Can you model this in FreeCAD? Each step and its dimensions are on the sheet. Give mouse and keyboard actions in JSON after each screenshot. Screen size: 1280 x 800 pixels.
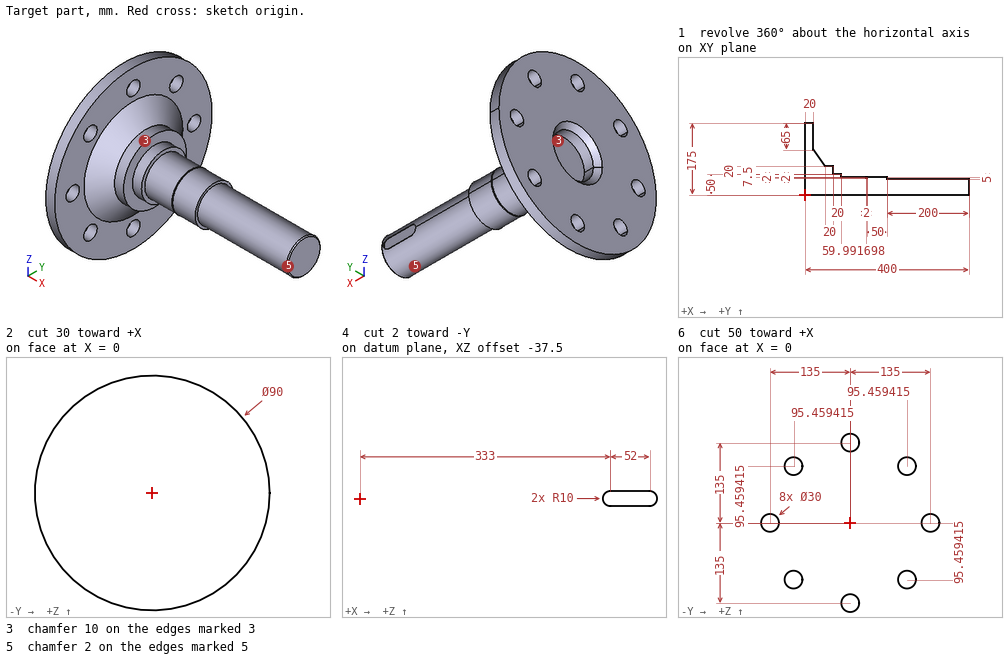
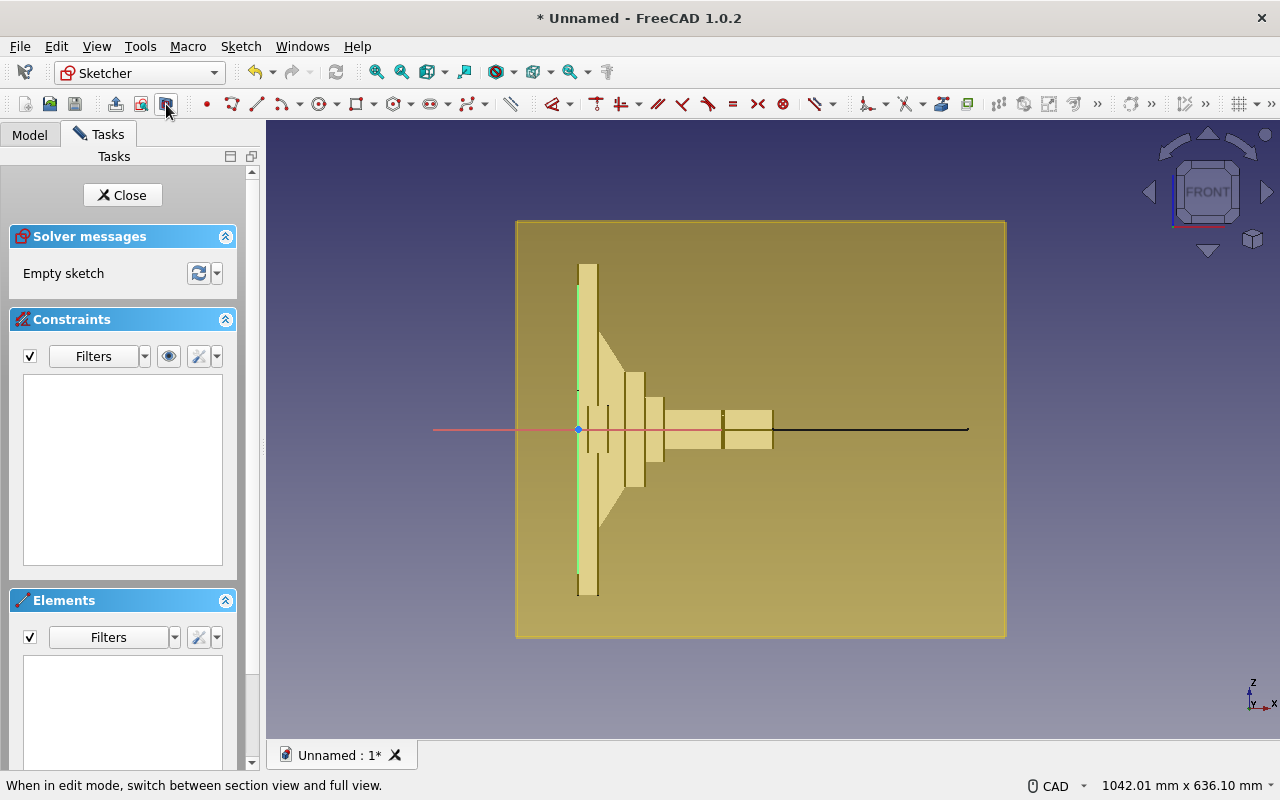
{"action": "scroll", "coordinate": [956, 430], "scroll_direction": "up", "scroll_amount": 11}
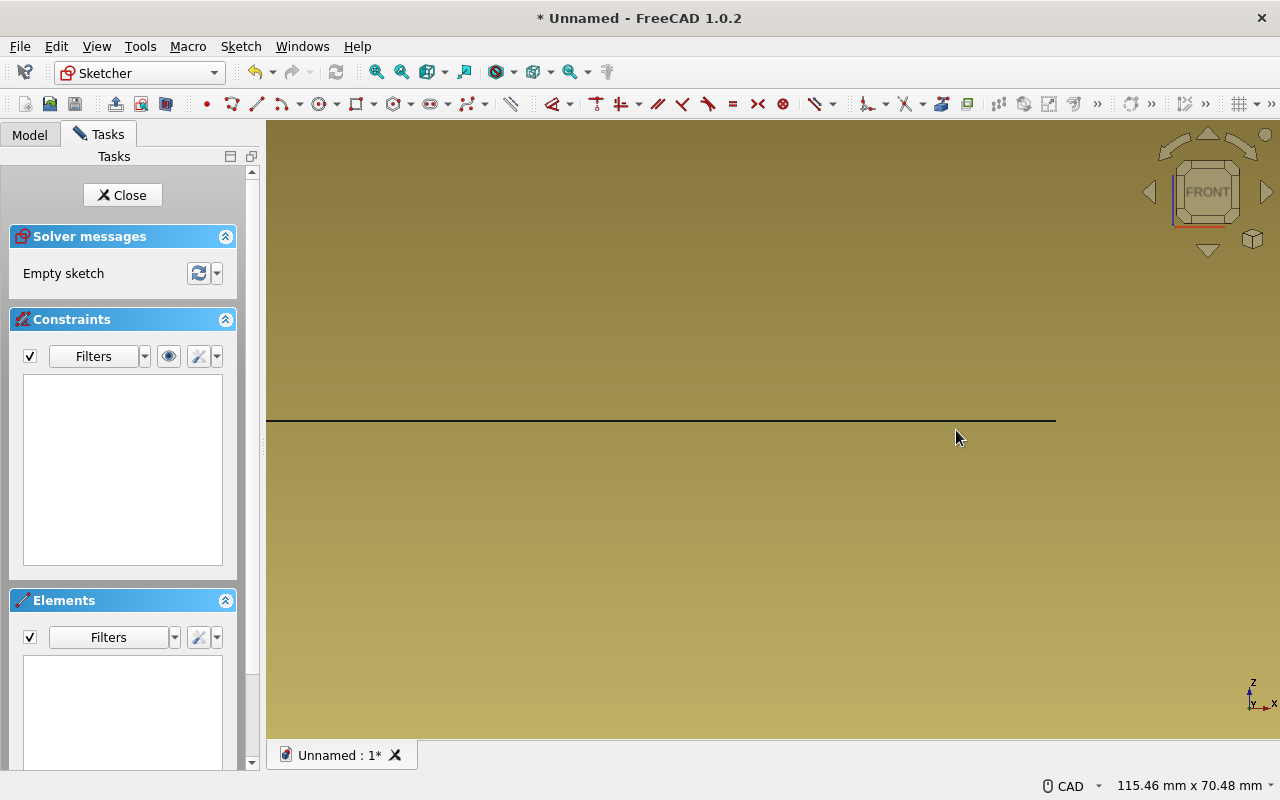
{"action": "left_click", "coordinate": [430, 104]}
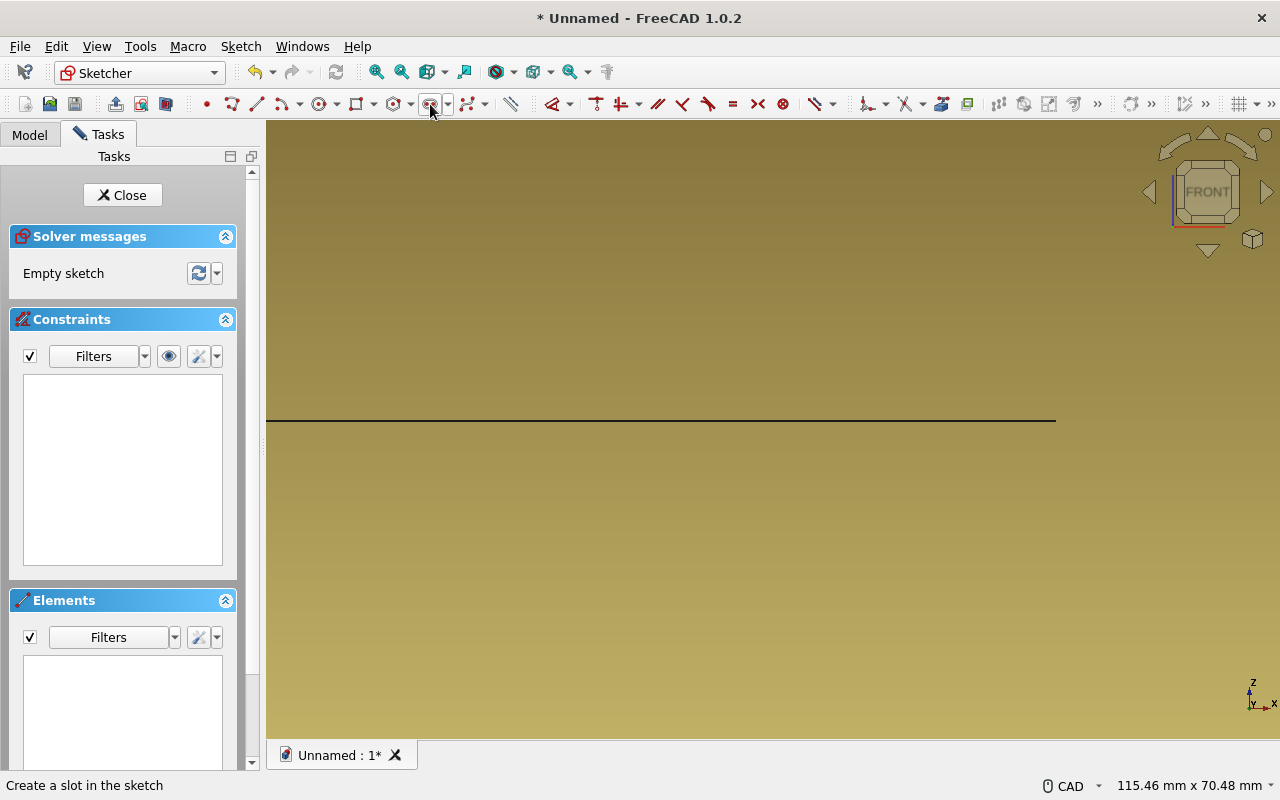
{"action": "left_click", "coordinate": [467, 421]}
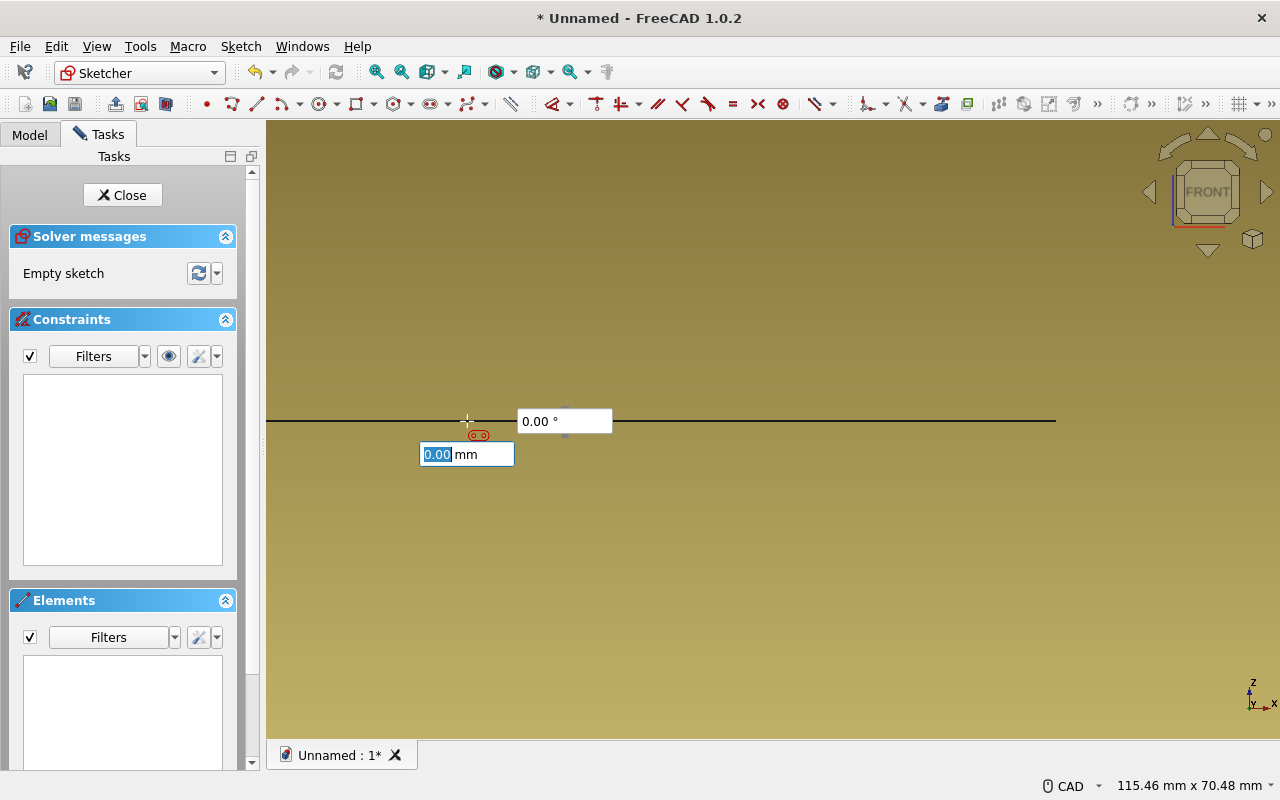
{"action": "left_click", "coordinate": [924, 412]}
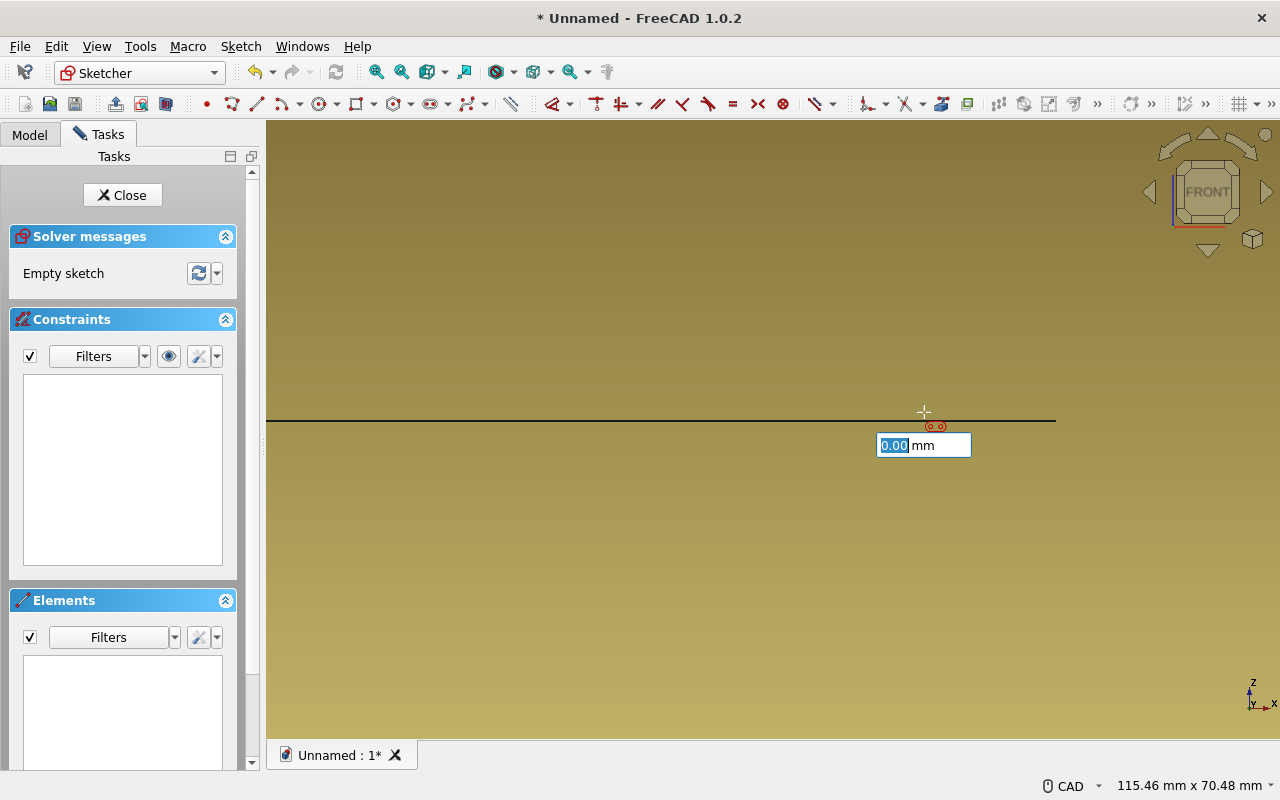
{"action": "left_click", "coordinate": [695, 509]}
{"action": "key", "text": "Escape"}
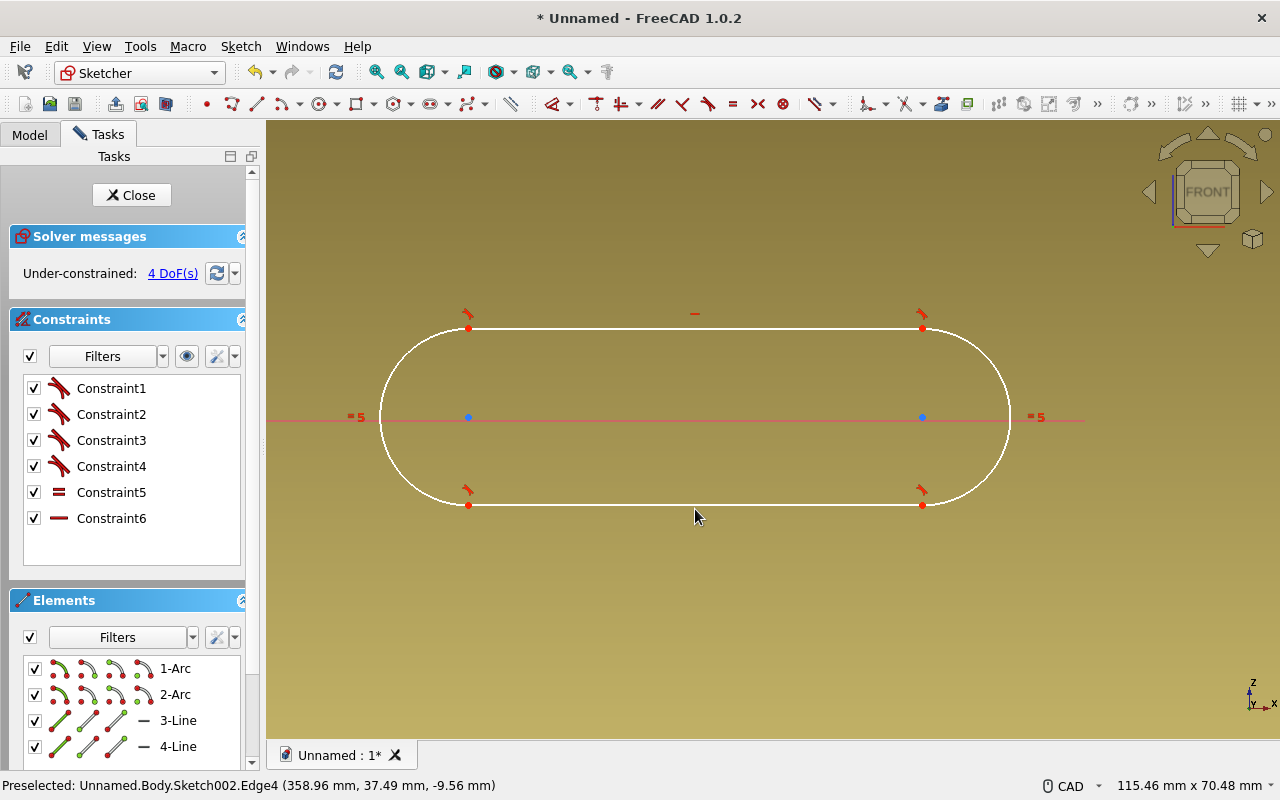
{"action": "left_click", "coordinate": [468, 417]}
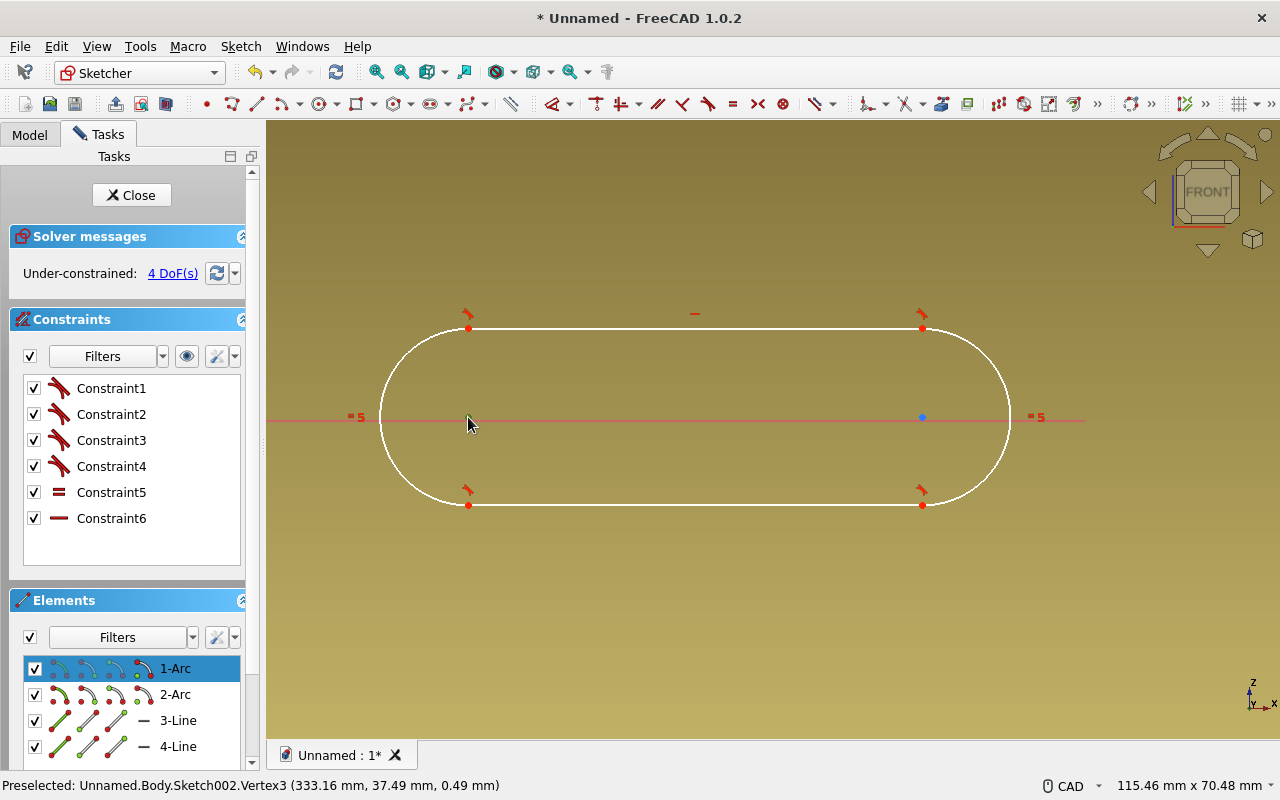
{"action": "left_click", "coordinate": [411, 421]}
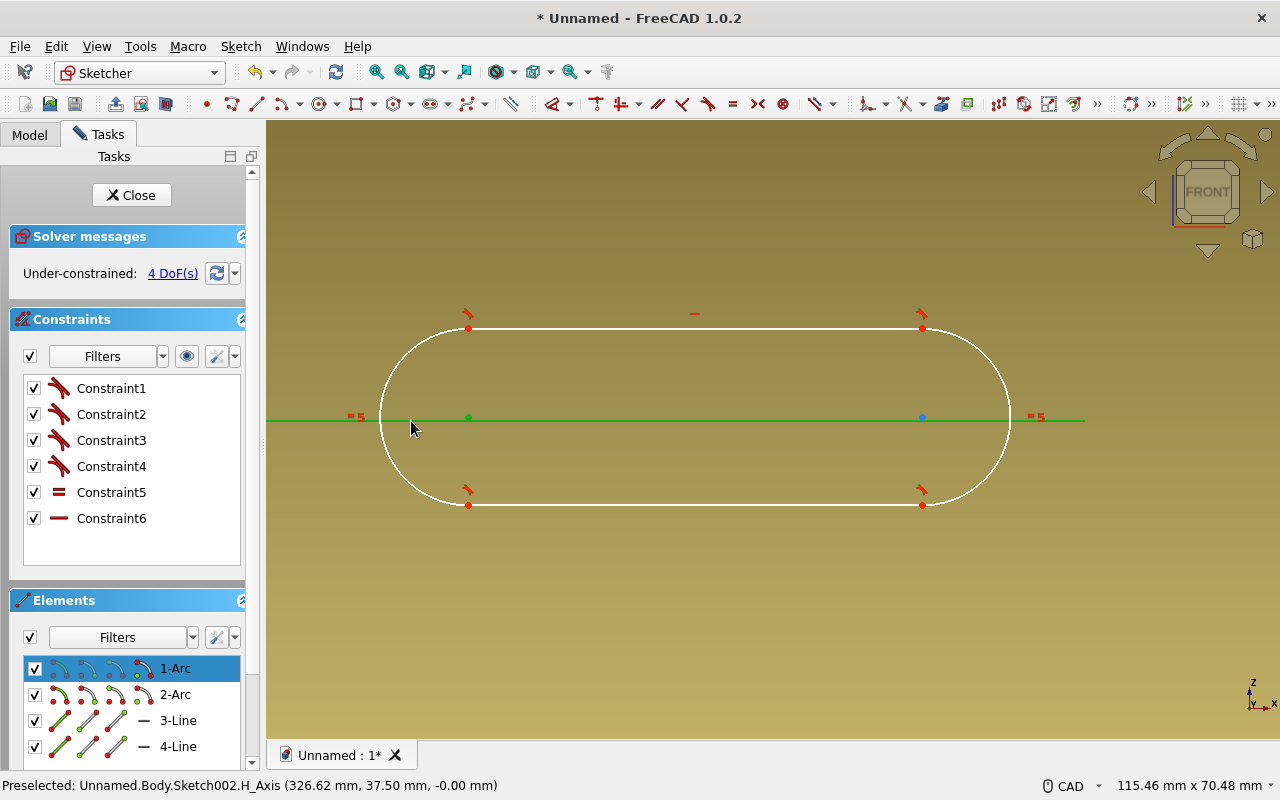
{"action": "left_click", "coordinate": [596, 104]}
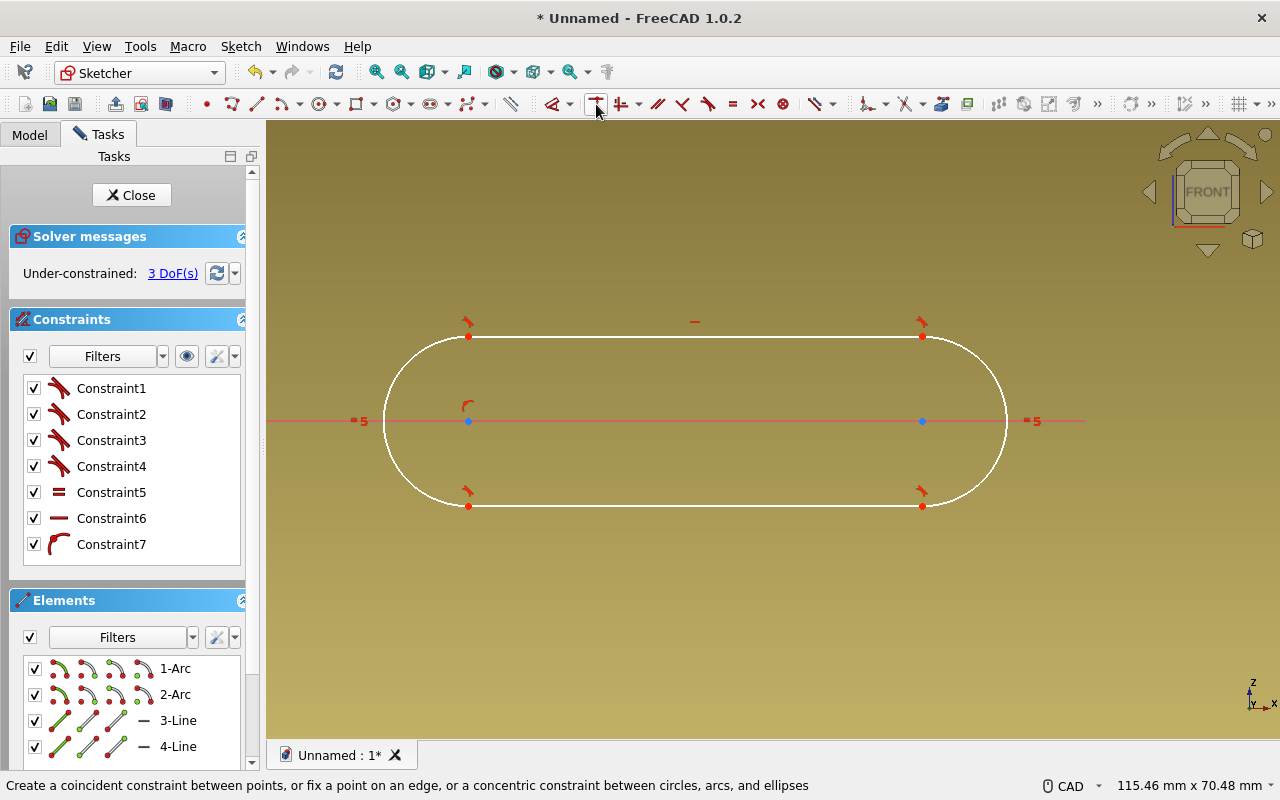
{"action": "left_click", "coordinate": [552, 104]}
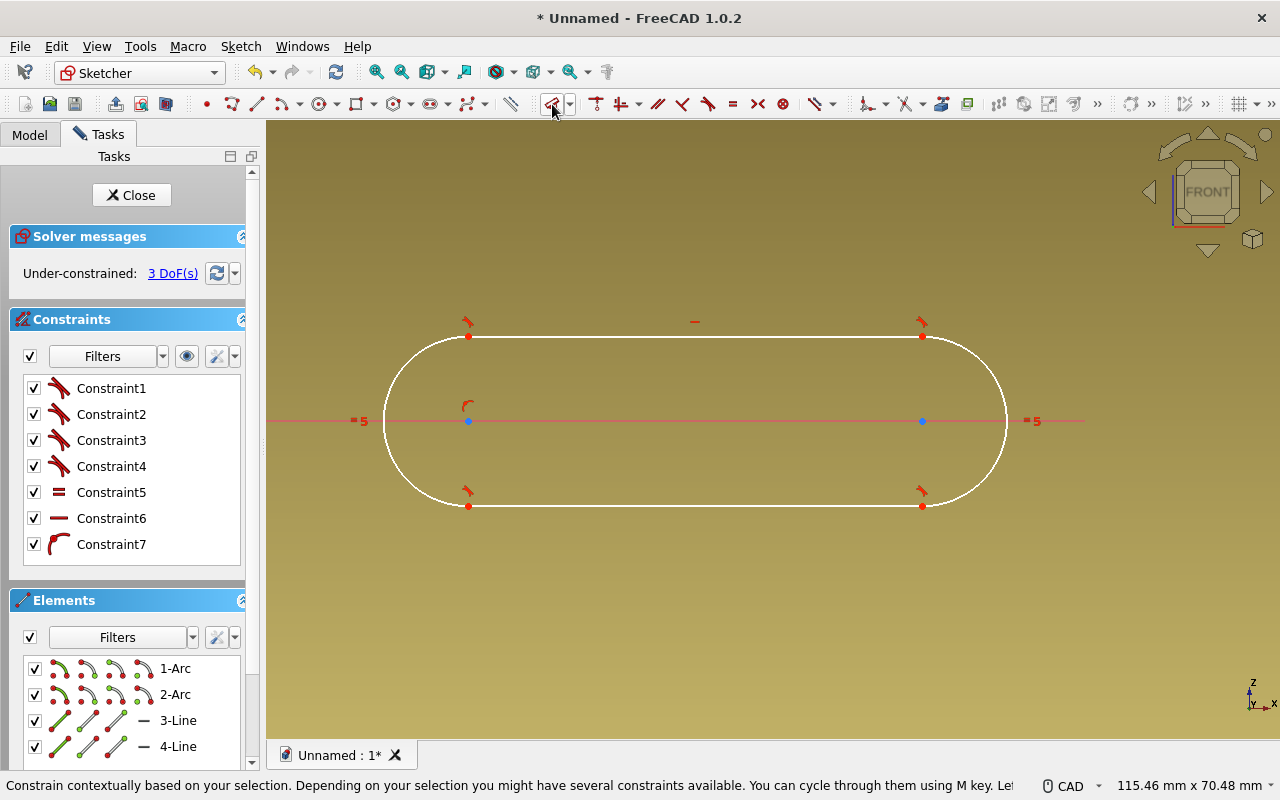
{"action": "left_click", "coordinate": [400, 372]}
{"action": "left_click", "coordinate": [374, 353]}